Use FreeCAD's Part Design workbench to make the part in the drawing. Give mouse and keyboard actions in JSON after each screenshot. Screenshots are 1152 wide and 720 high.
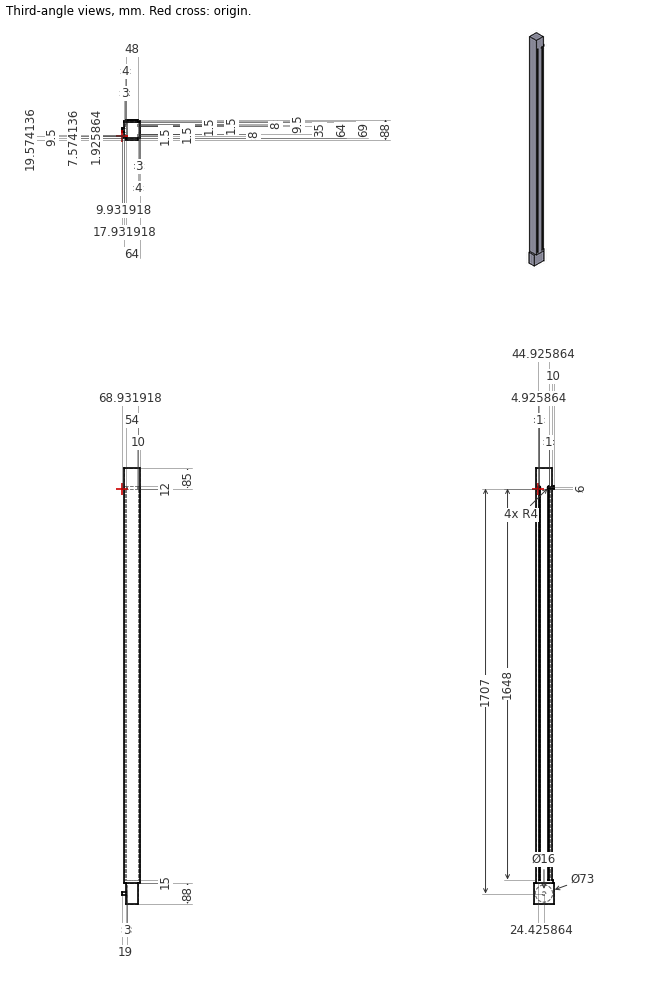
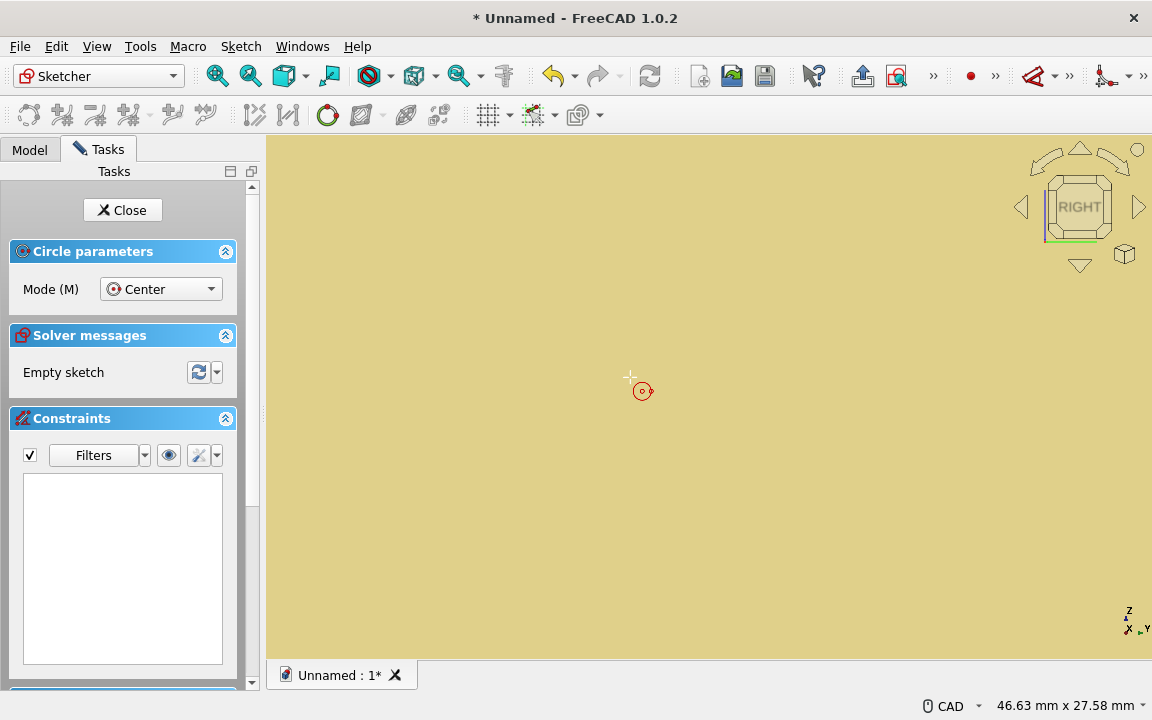
{"action": "left_click", "coordinate": [638, 390]}
{"action": "mouse_move", "coordinate": [745, 283]}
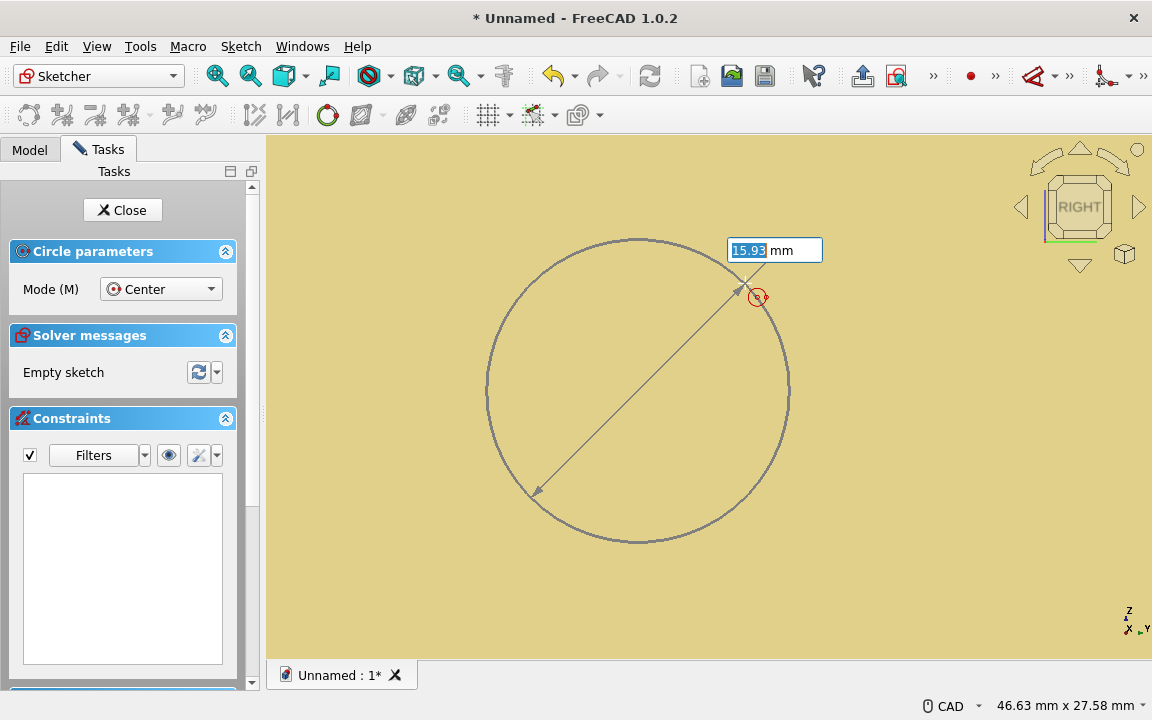
{"action": "type", "text": "16"}
{"action": "key", "text": "Return"}
{"action": "key", "text": "Escape"}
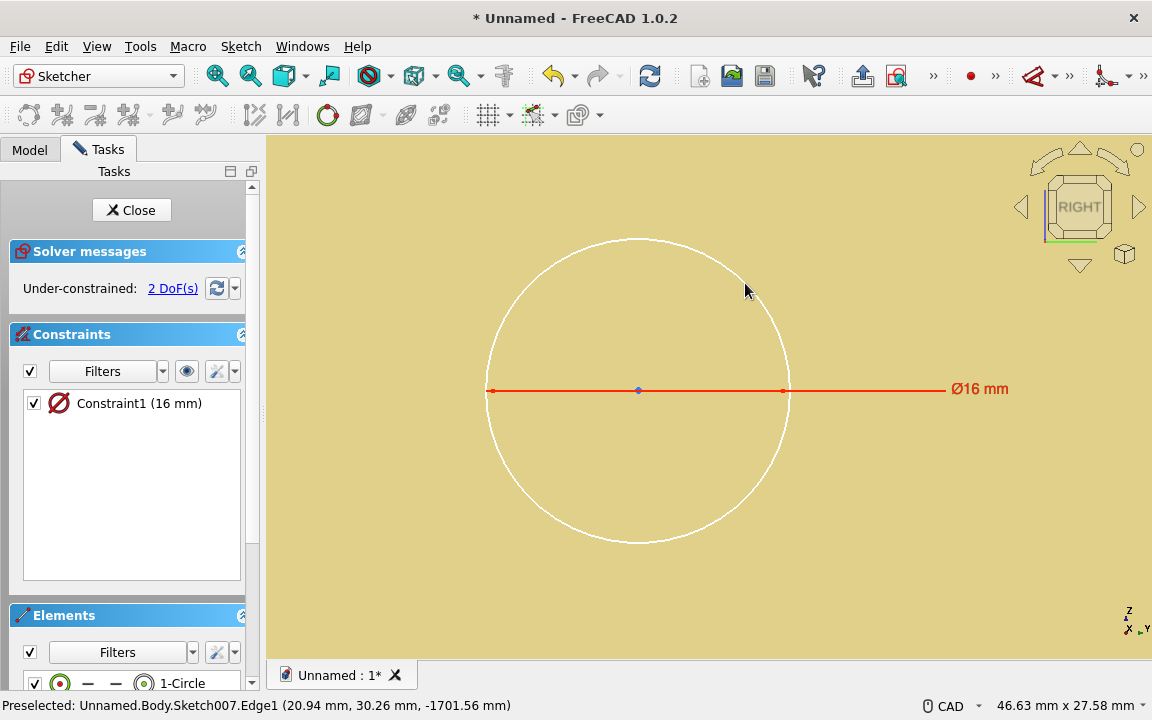
{"action": "left_click", "coordinate": [1032, 76]}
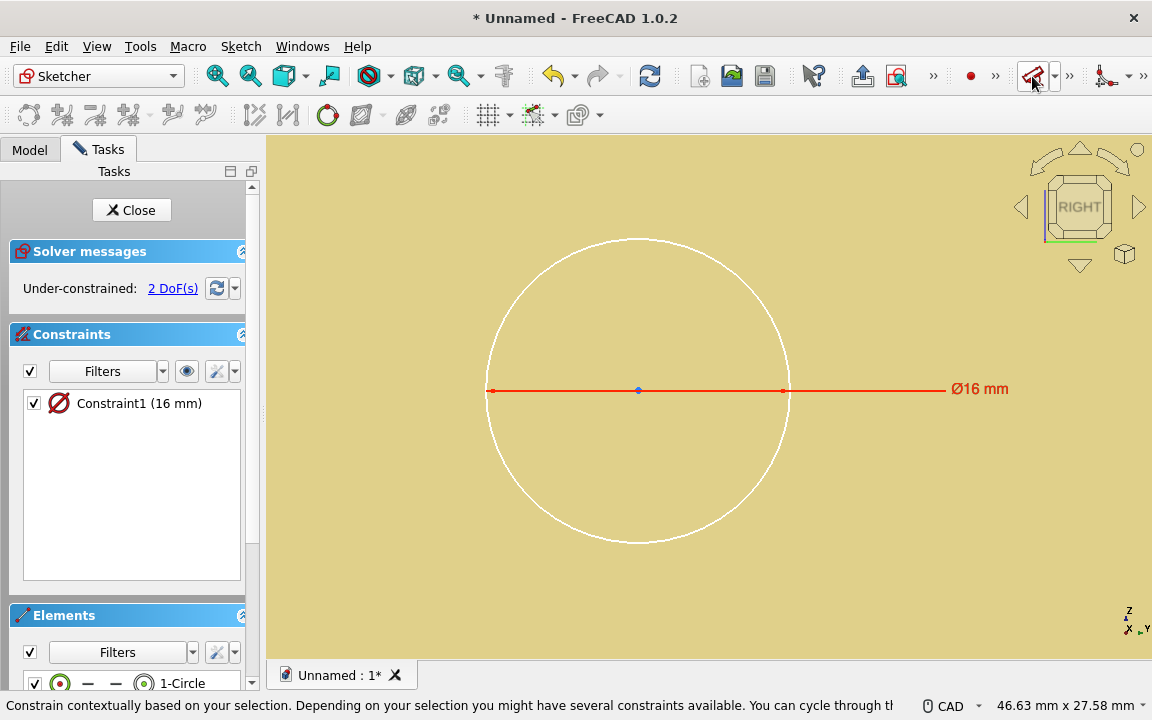
{"action": "left_click", "coordinate": [638, 391]}
{"action": "left_click", "coordinate": [672, 277]}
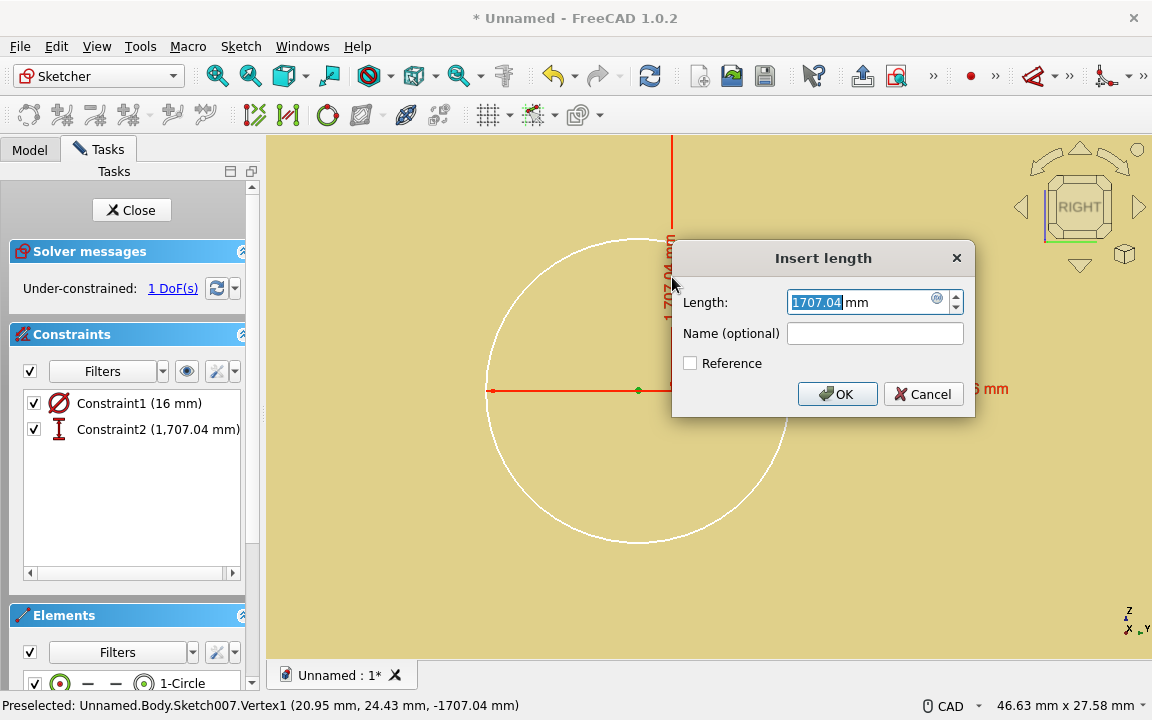
{"action": "type", "text": "1707"}
{"action": "key", "text": "Return"}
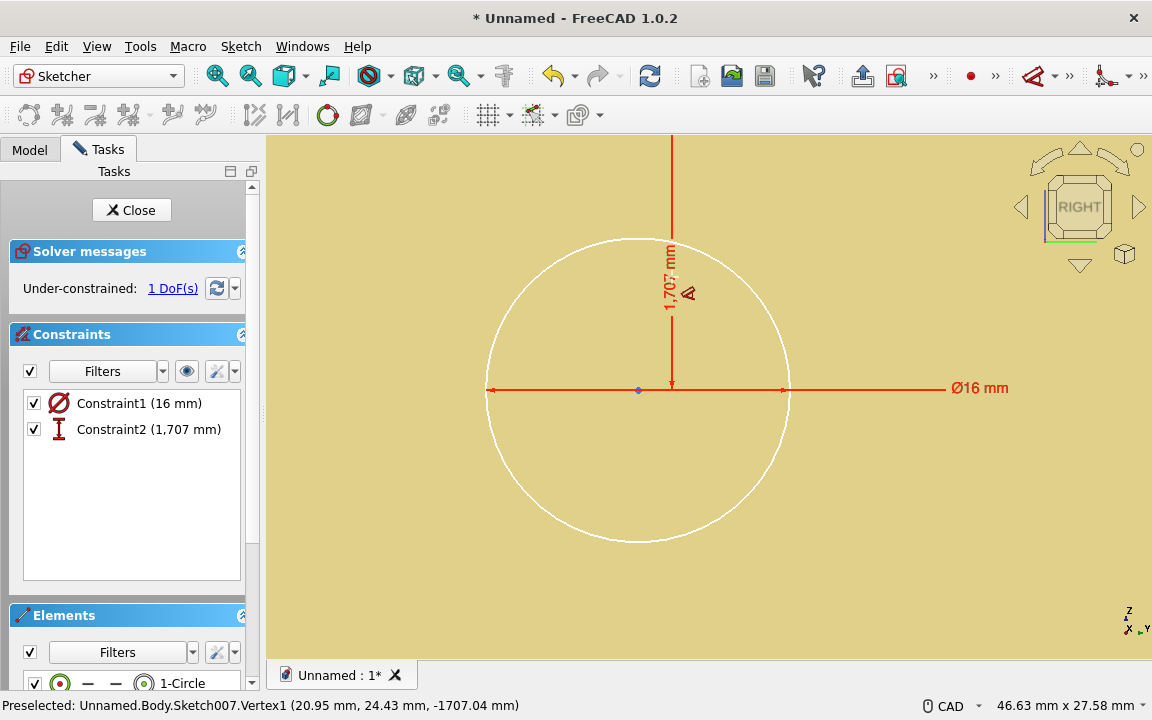
{"action": "left_click", "coordinate": [638, 390]}
{"action": "left_click", "coordinate": [466, 424]}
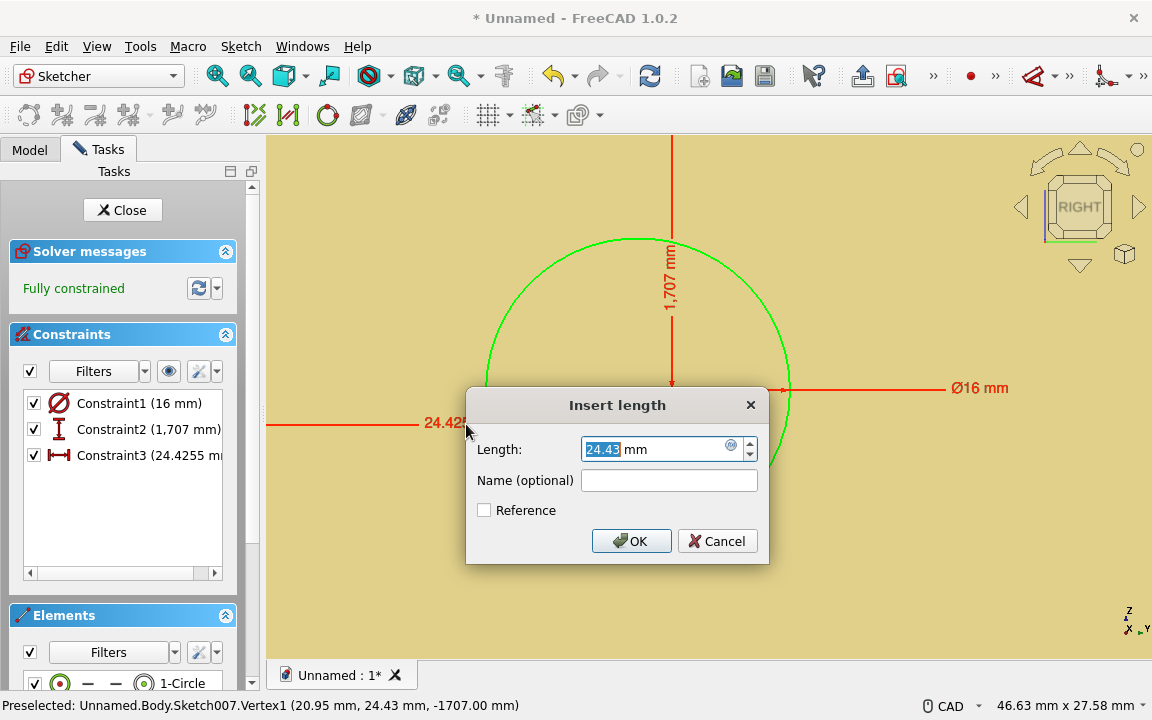
{"action": "type", "text": "24.425864"}
{"action": "key", "text": "Return"}
{"action": "key", "text": "Escape"}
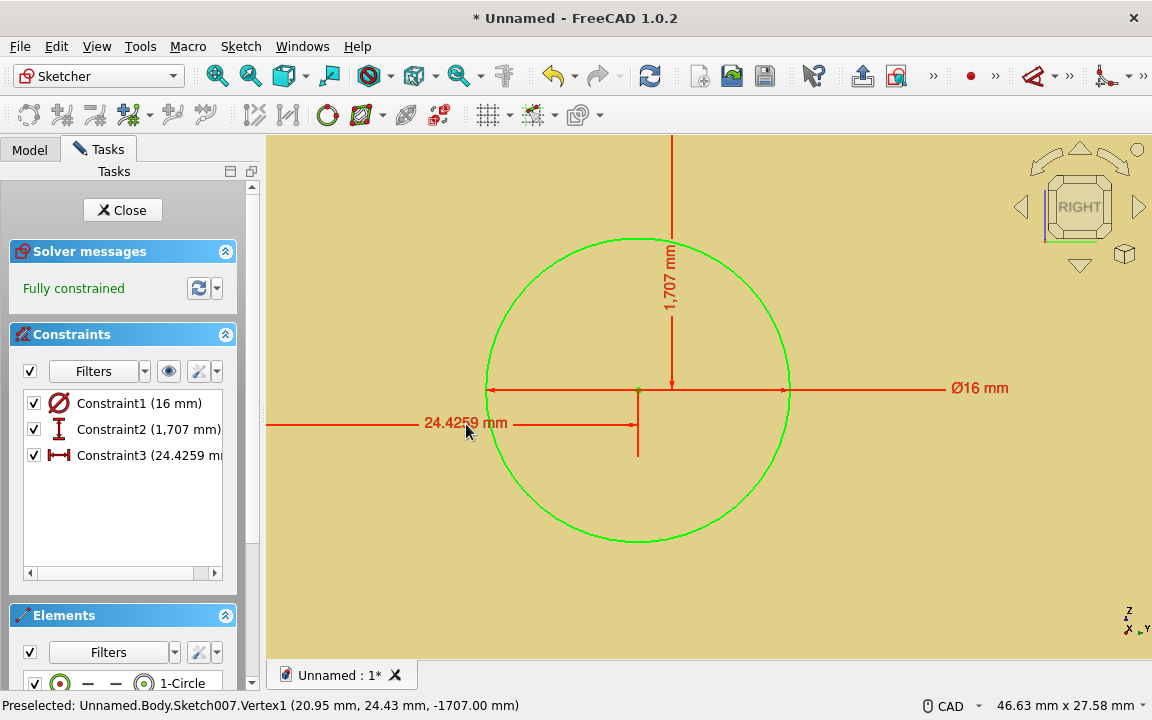
{"action": "left_click", "coordinate": [123, 210]}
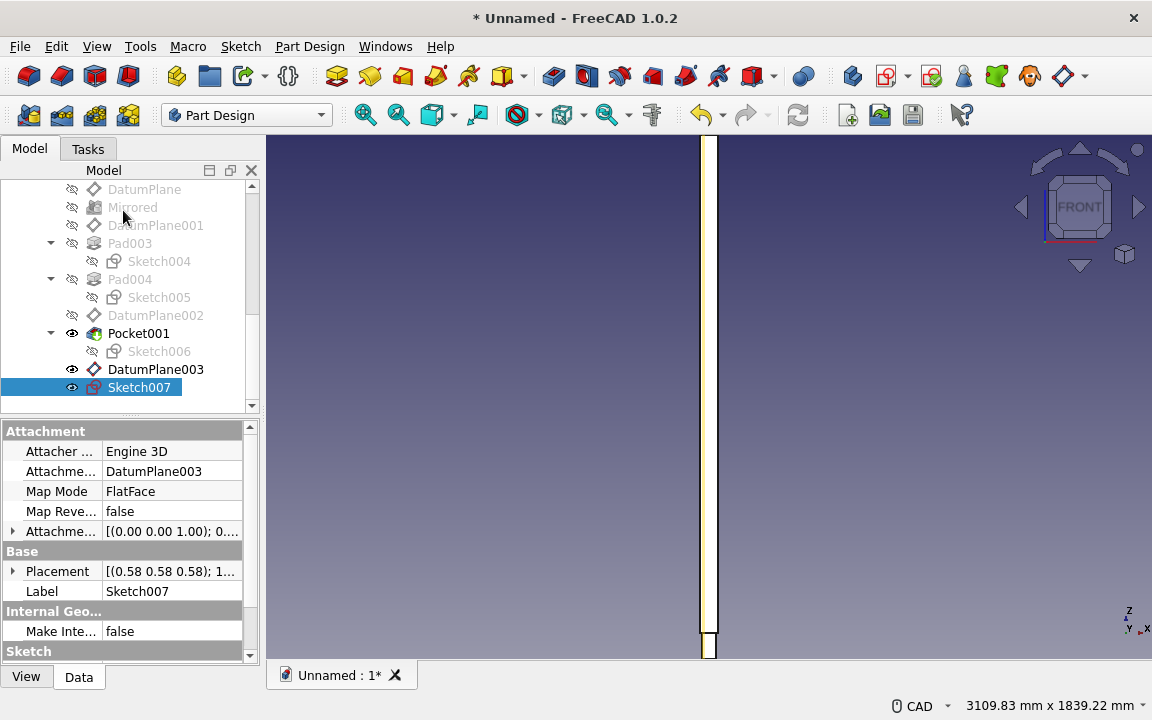
{"action": "left_click", "coordinate": [337, 76]}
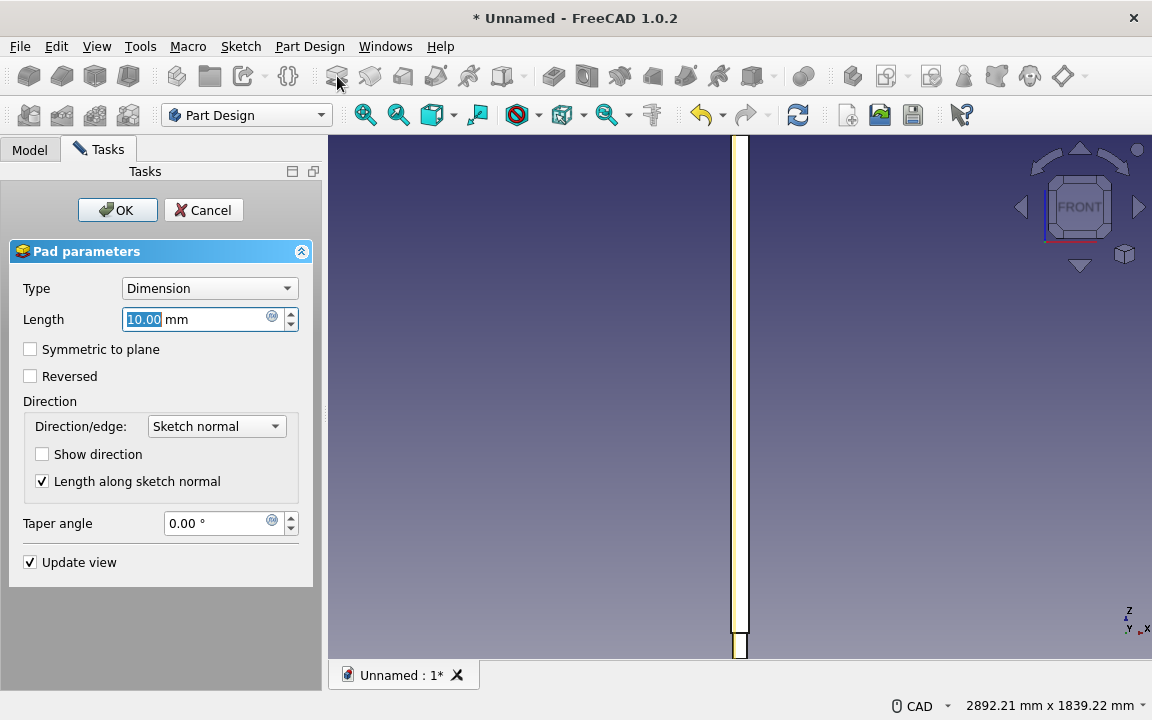
{"action": "type", "text": "19"}
{"action": "key", "text": "Tab"}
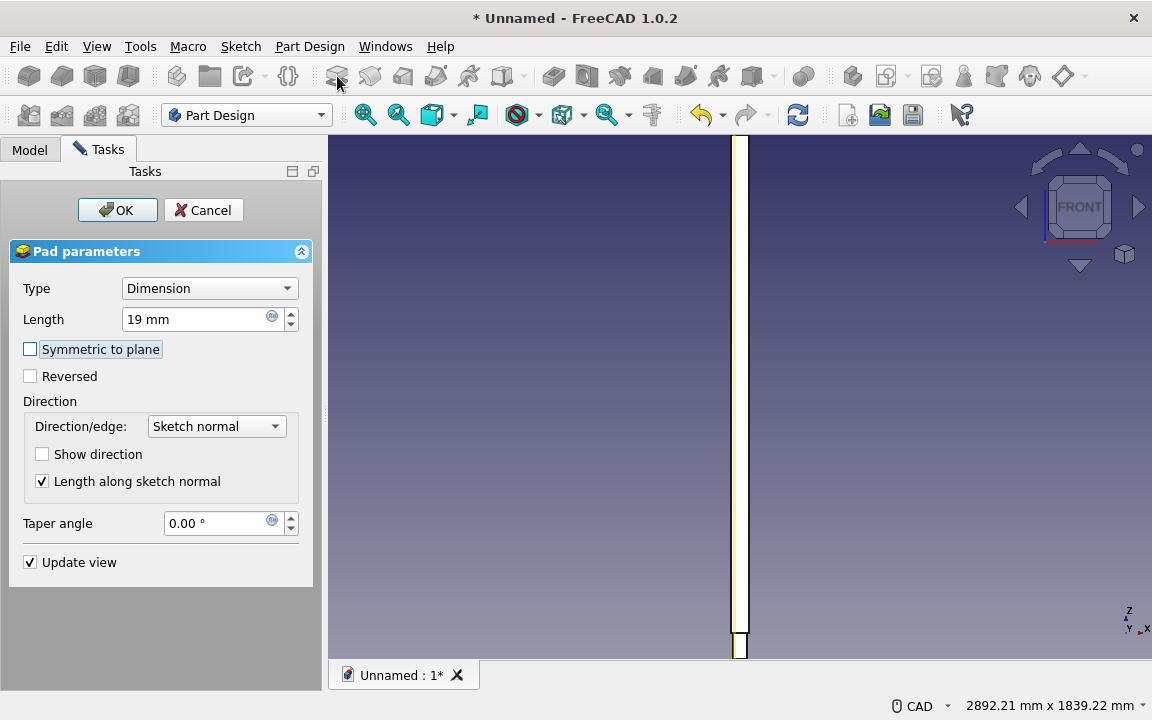
{"action": "left_click", "coordinate": [31, 376]}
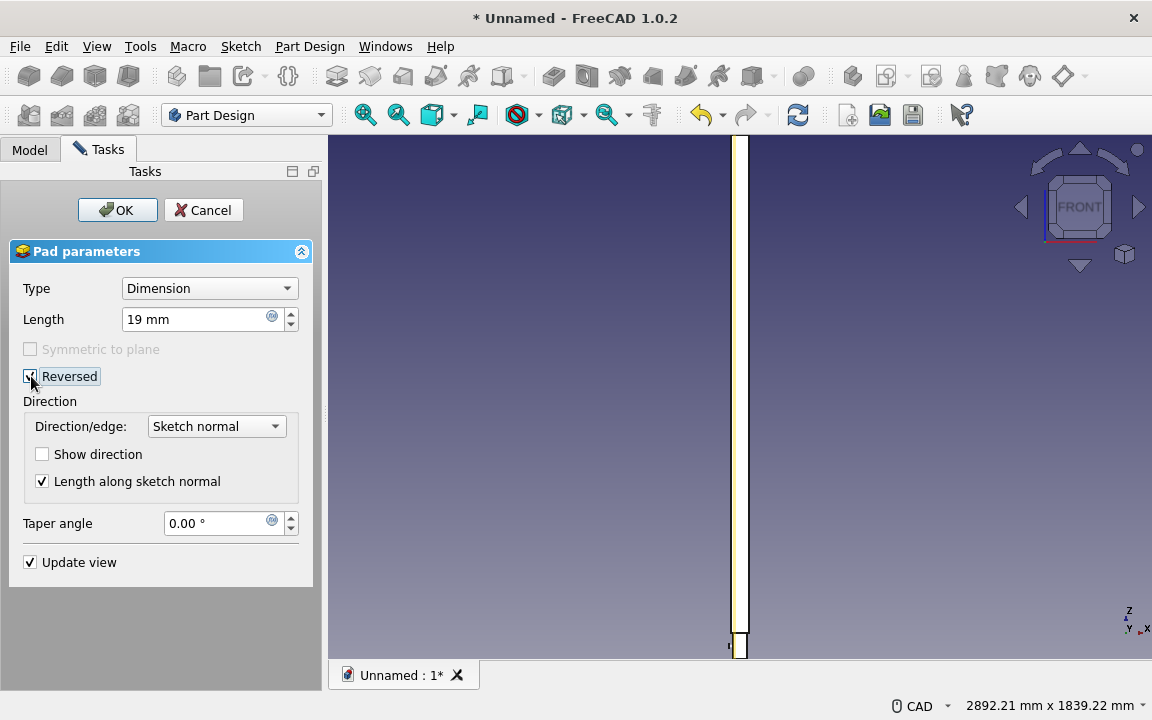
{"action": "left_click", "coordinate": [118, 210]}